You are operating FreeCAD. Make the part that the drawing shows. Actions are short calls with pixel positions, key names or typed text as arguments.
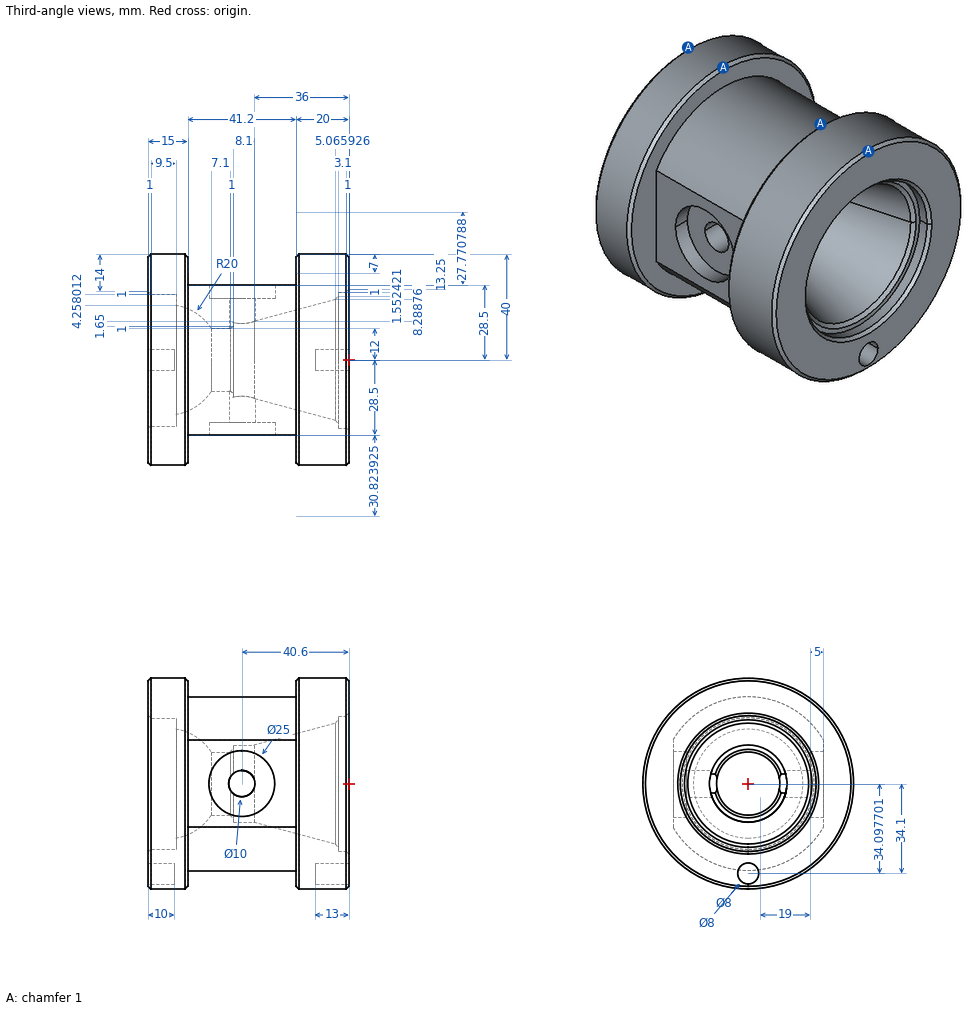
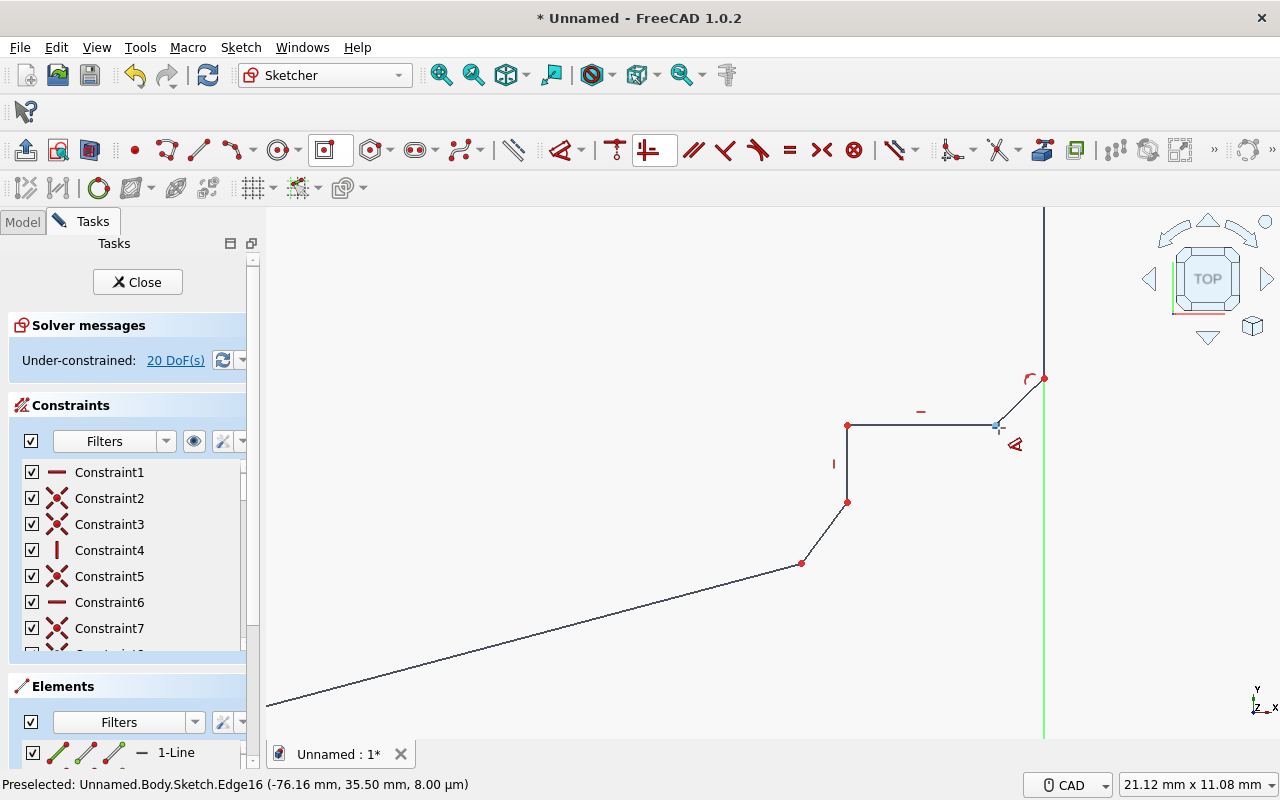
click(996, 425)
click(1009, 391)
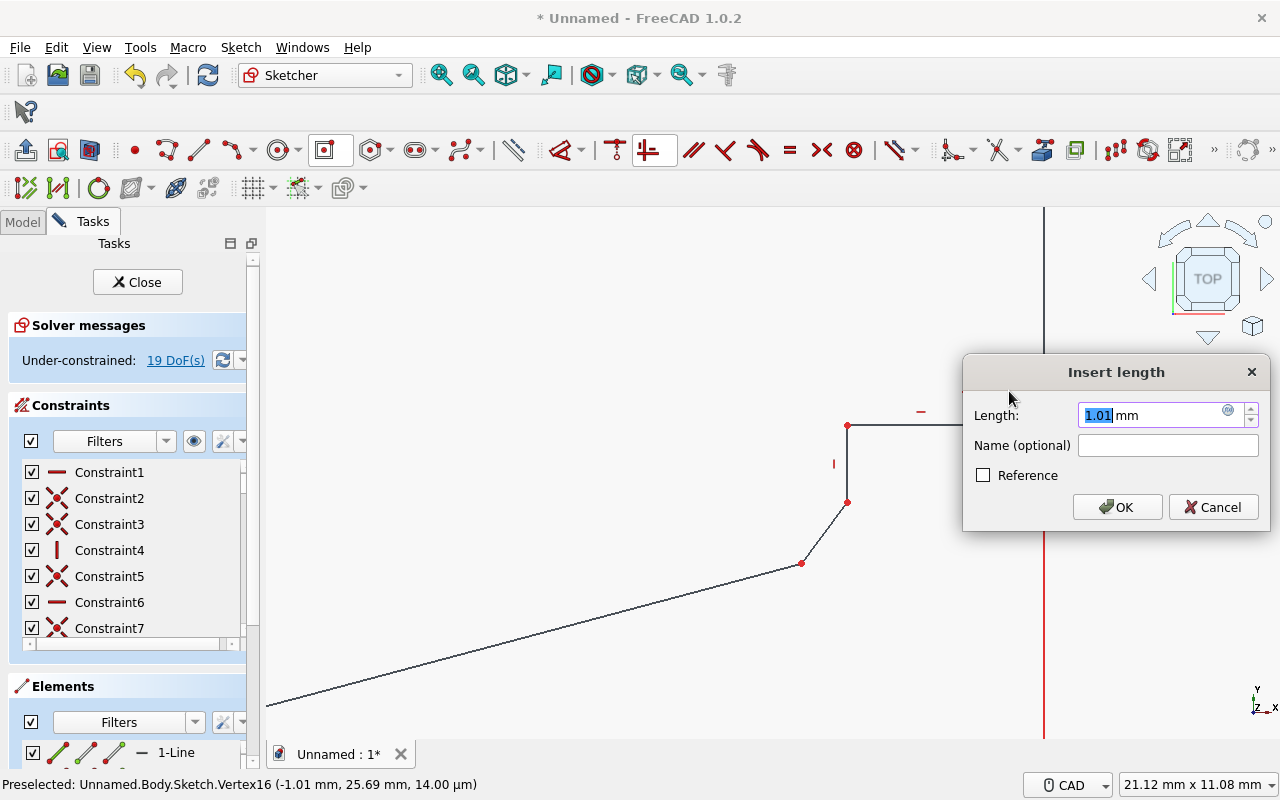
text(1)
key(Return)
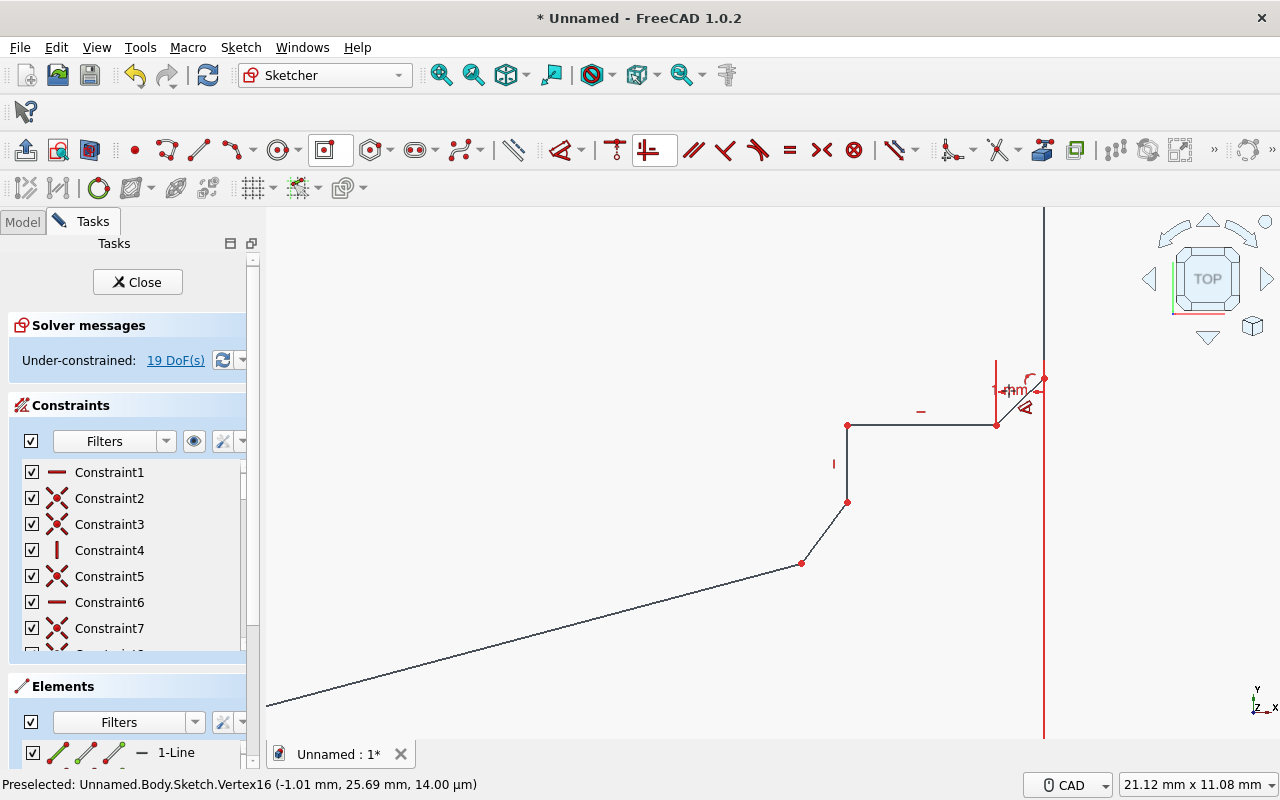
scroll(999, 428, down, 9)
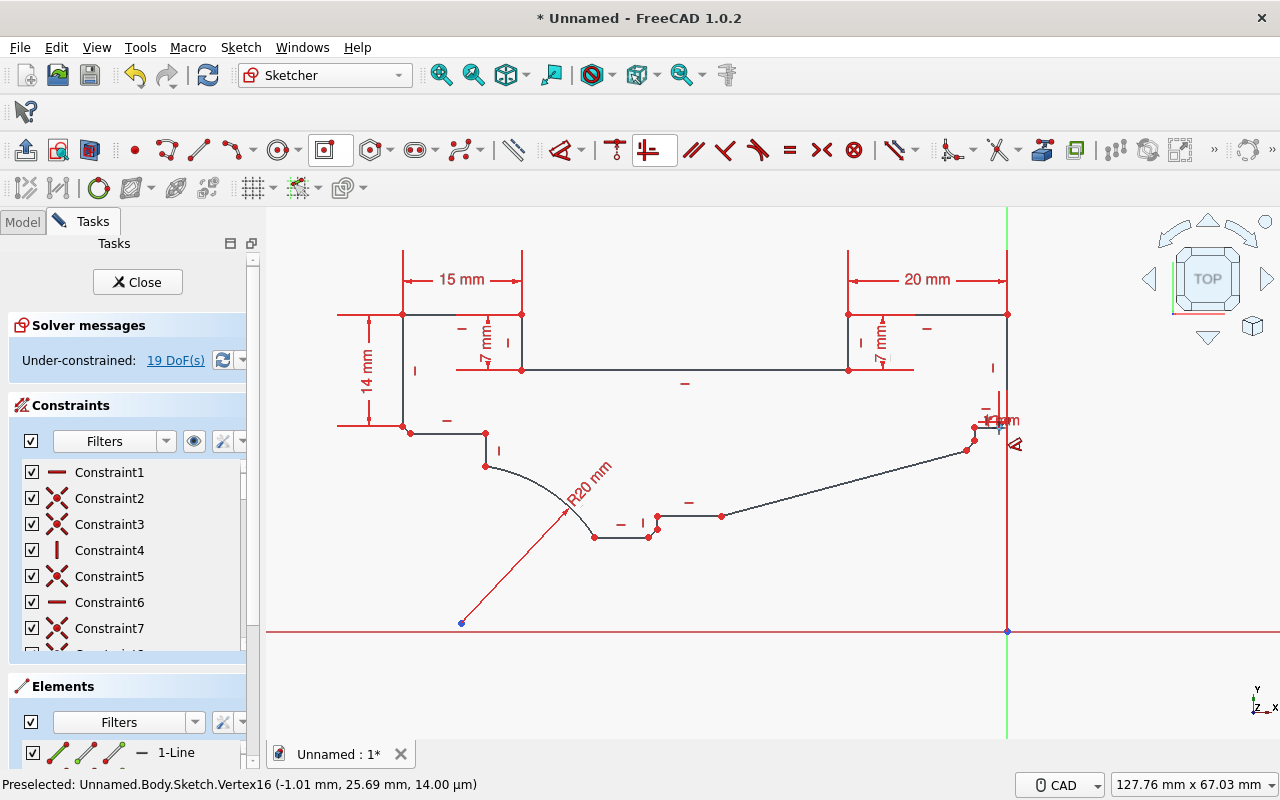
scroll(651, 535, up, 9)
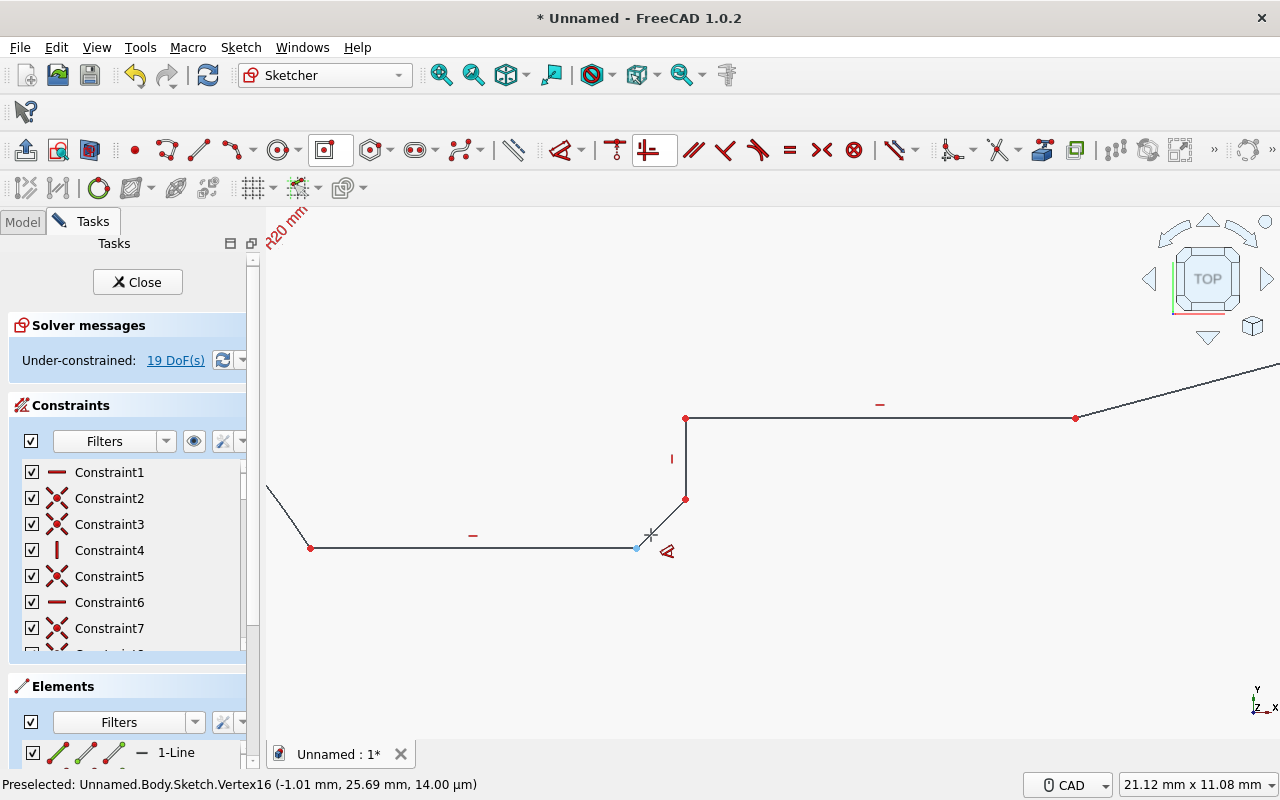
click(652, 534)
click(661, 582)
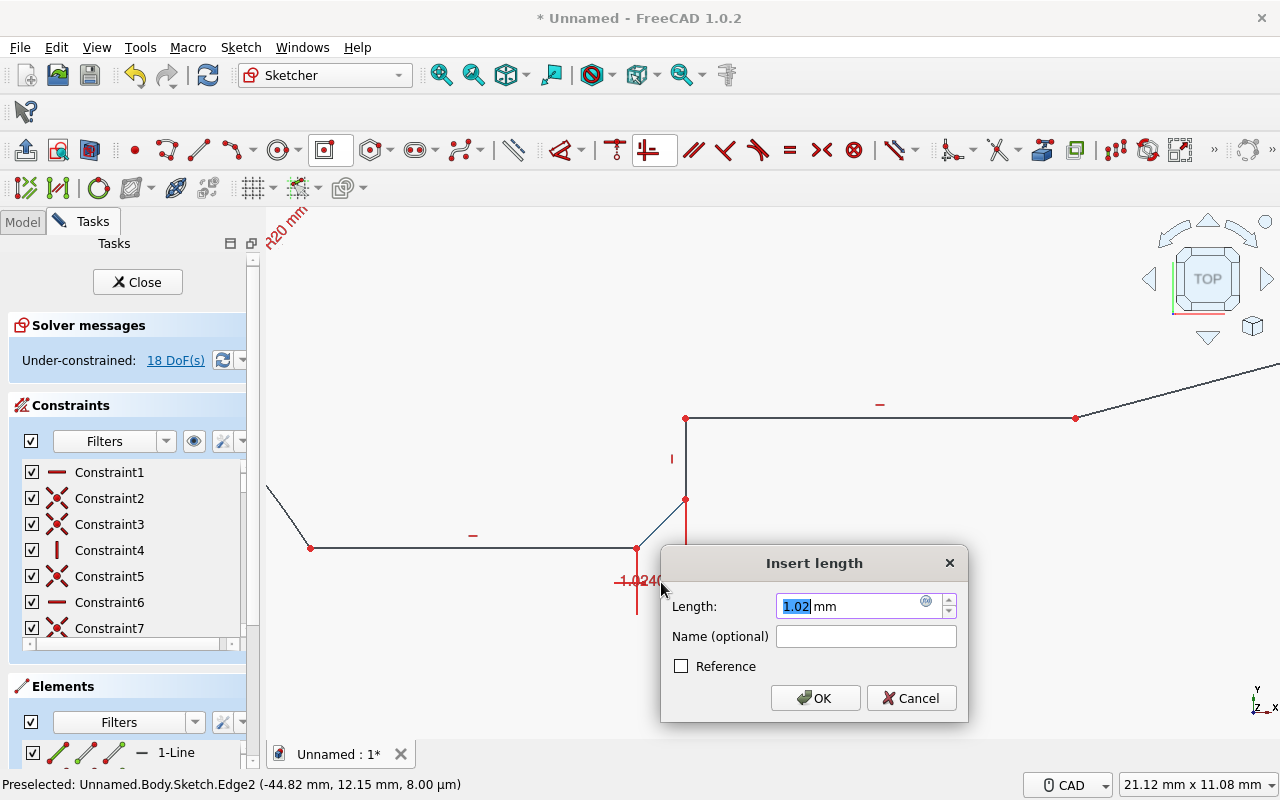
text(1)
key(Return)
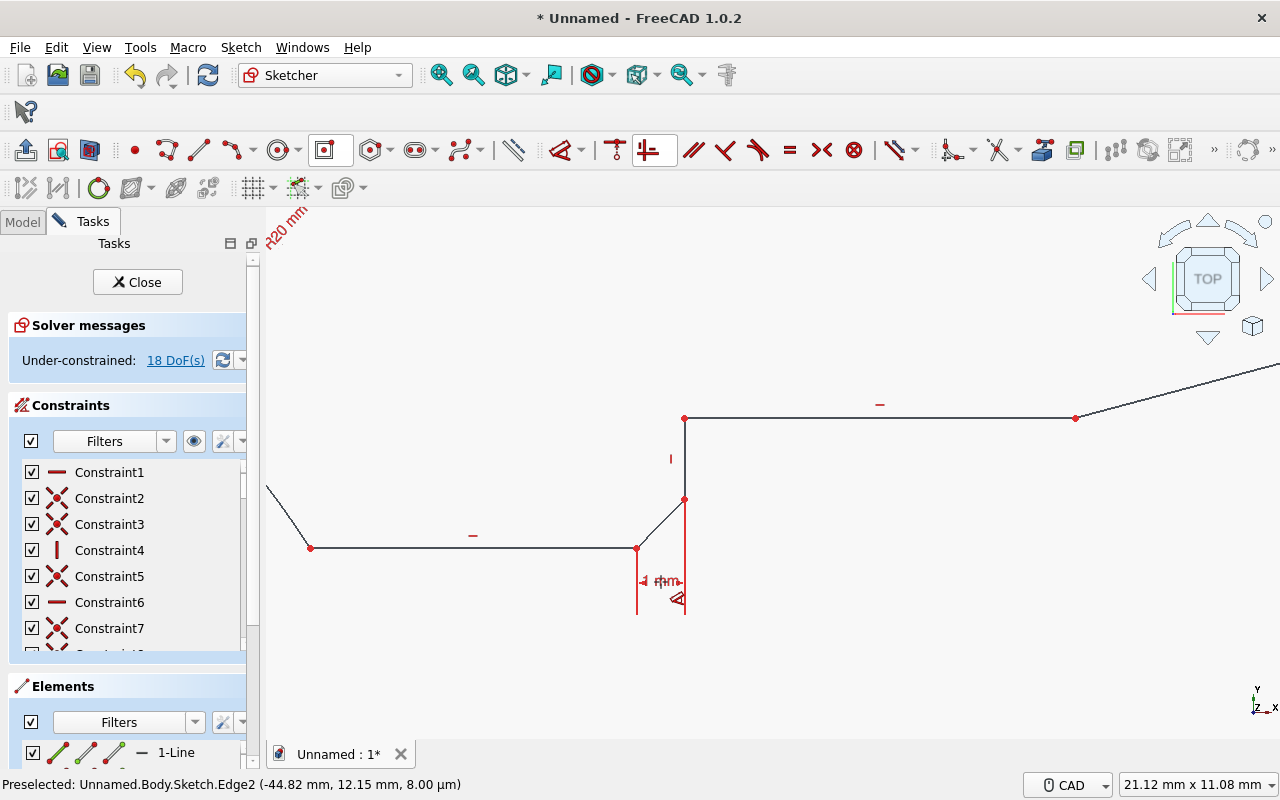
click(651, 534)
click(603, 524)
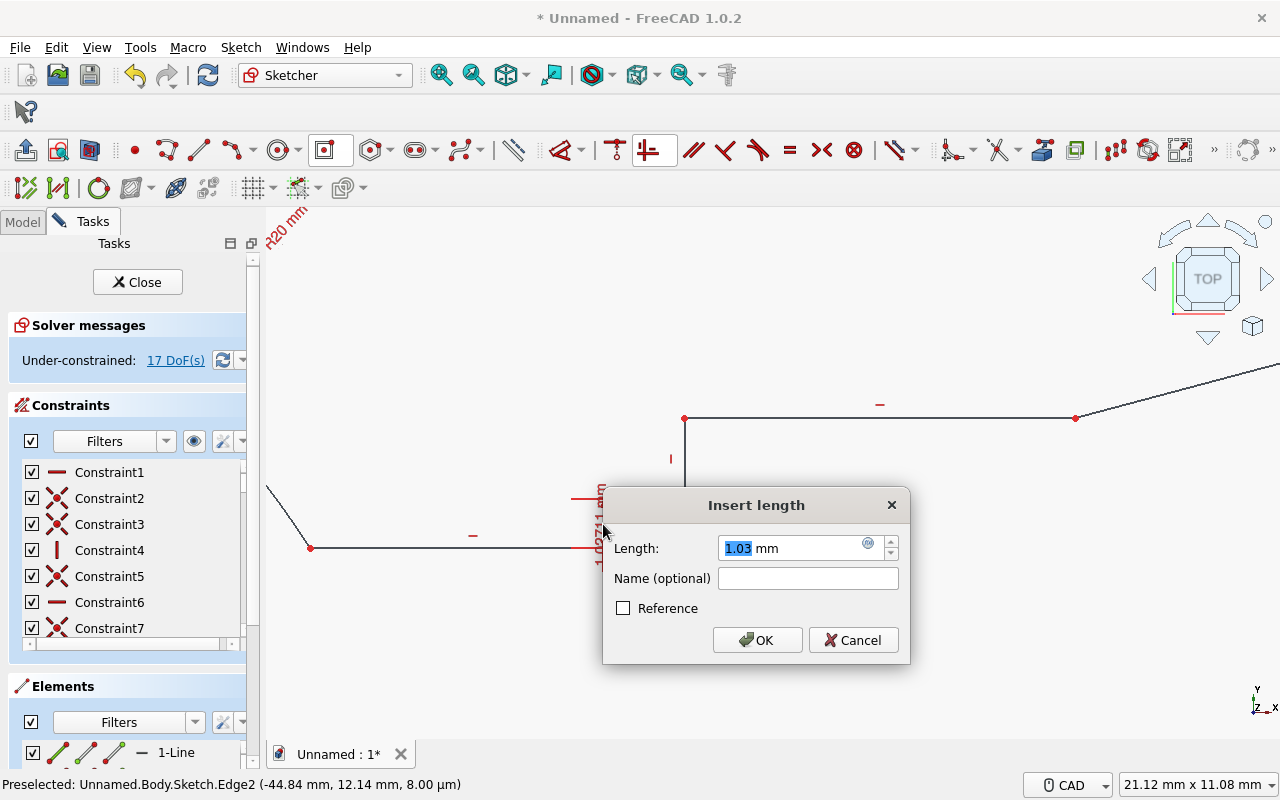
text(1)
key(Return)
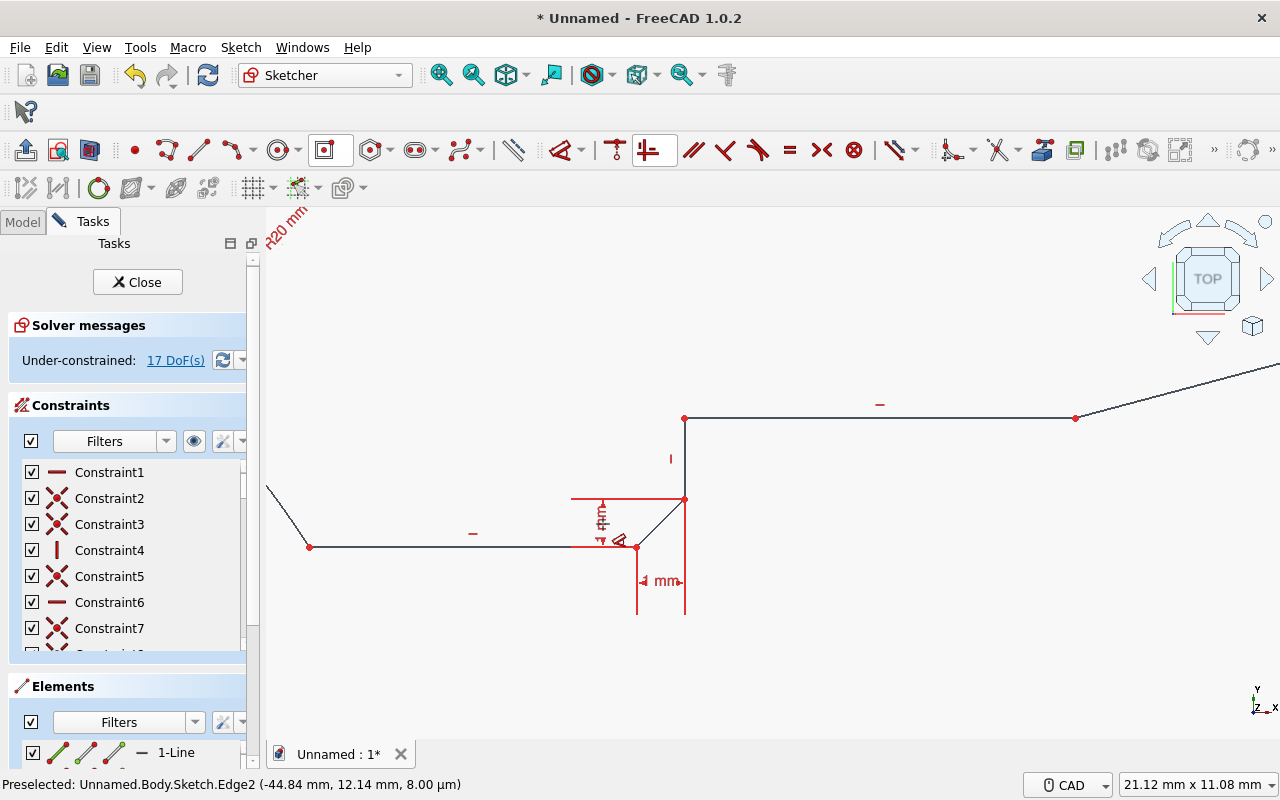
scroll(651, 536, down, 9)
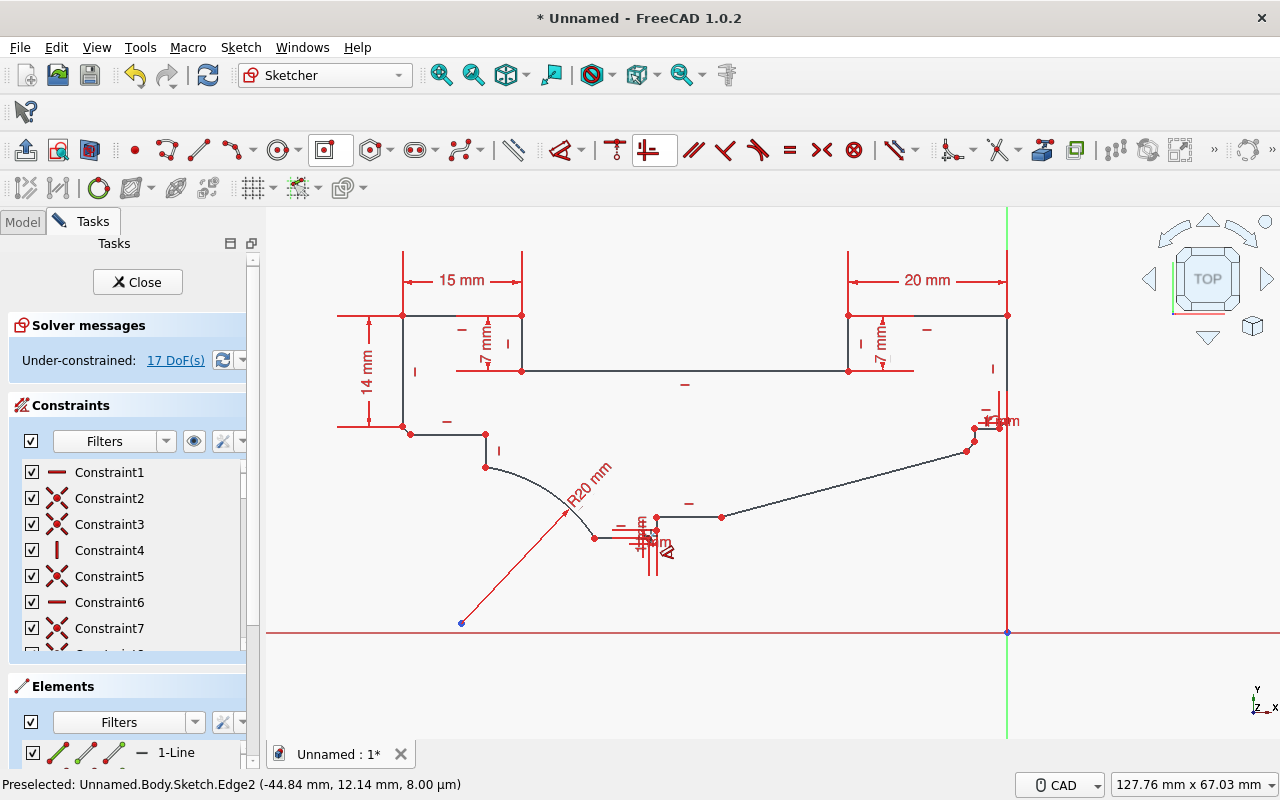
scroll(1002, 426, up, 9)